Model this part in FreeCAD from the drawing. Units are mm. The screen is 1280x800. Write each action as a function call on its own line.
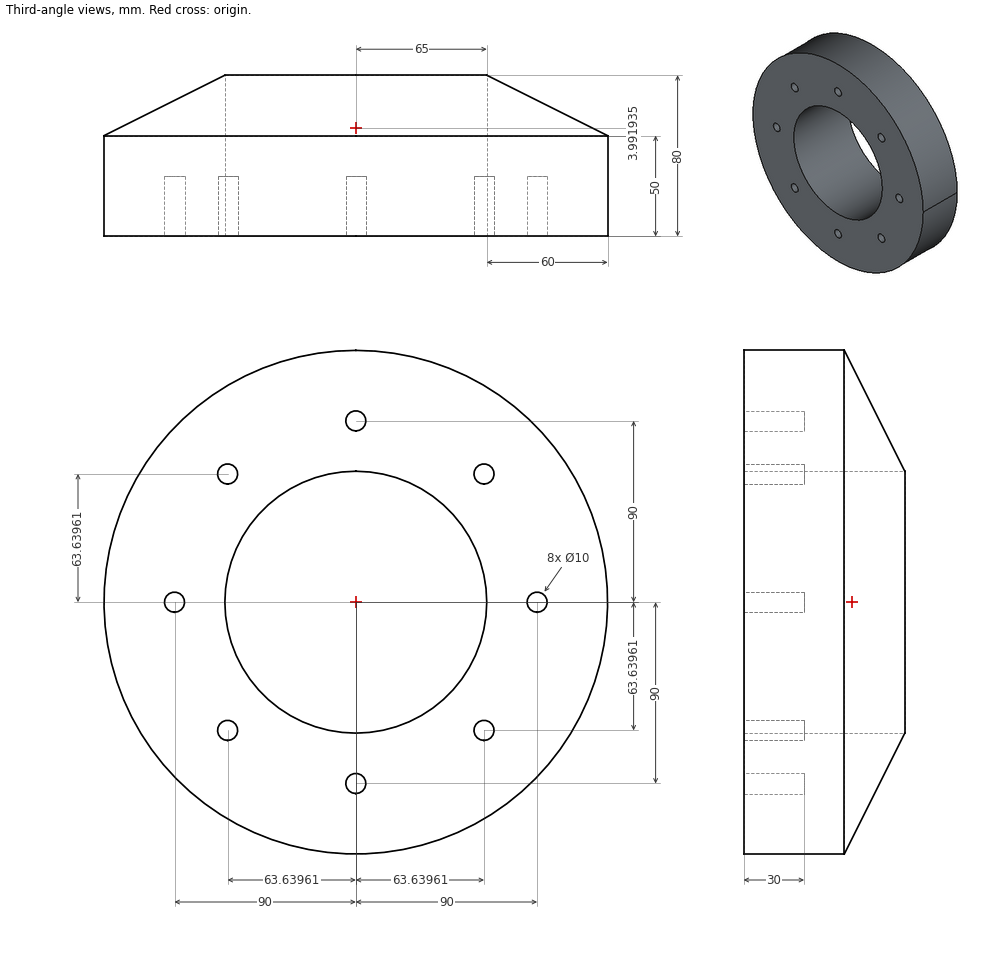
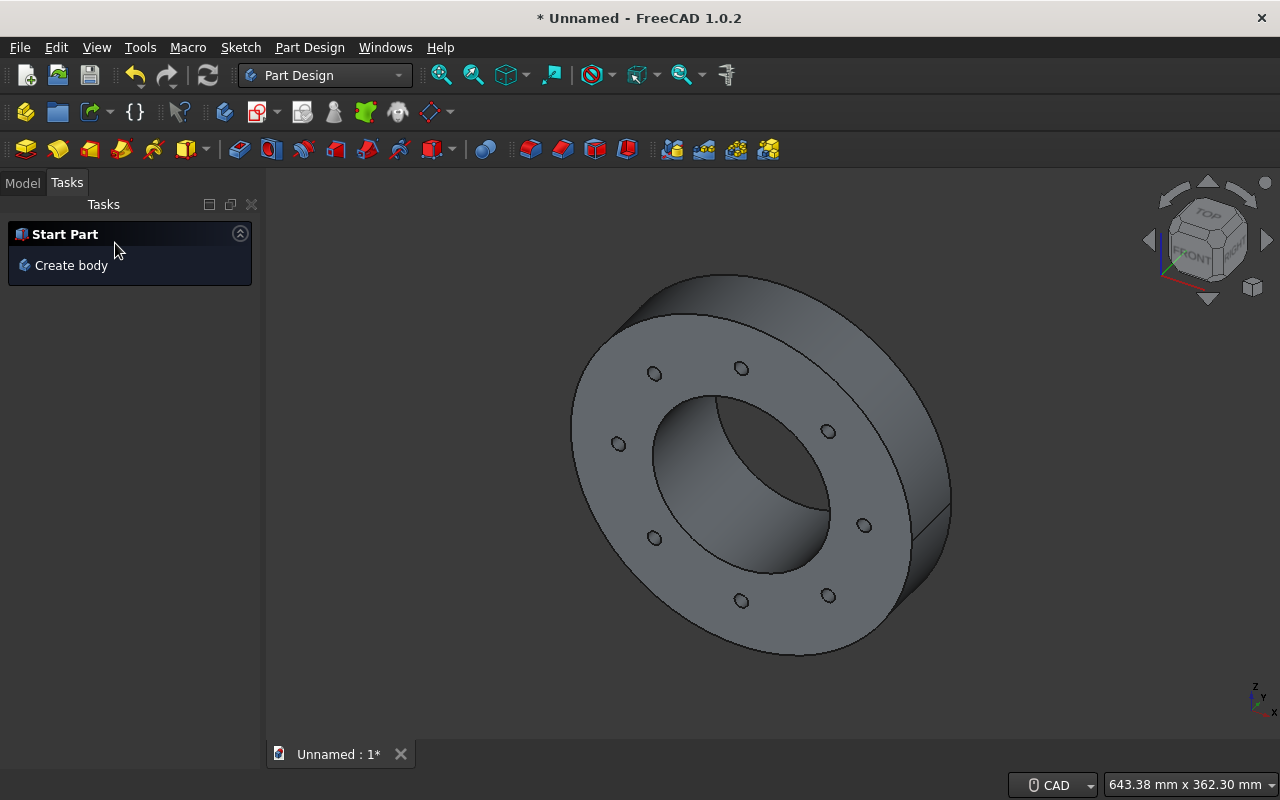
key(0)